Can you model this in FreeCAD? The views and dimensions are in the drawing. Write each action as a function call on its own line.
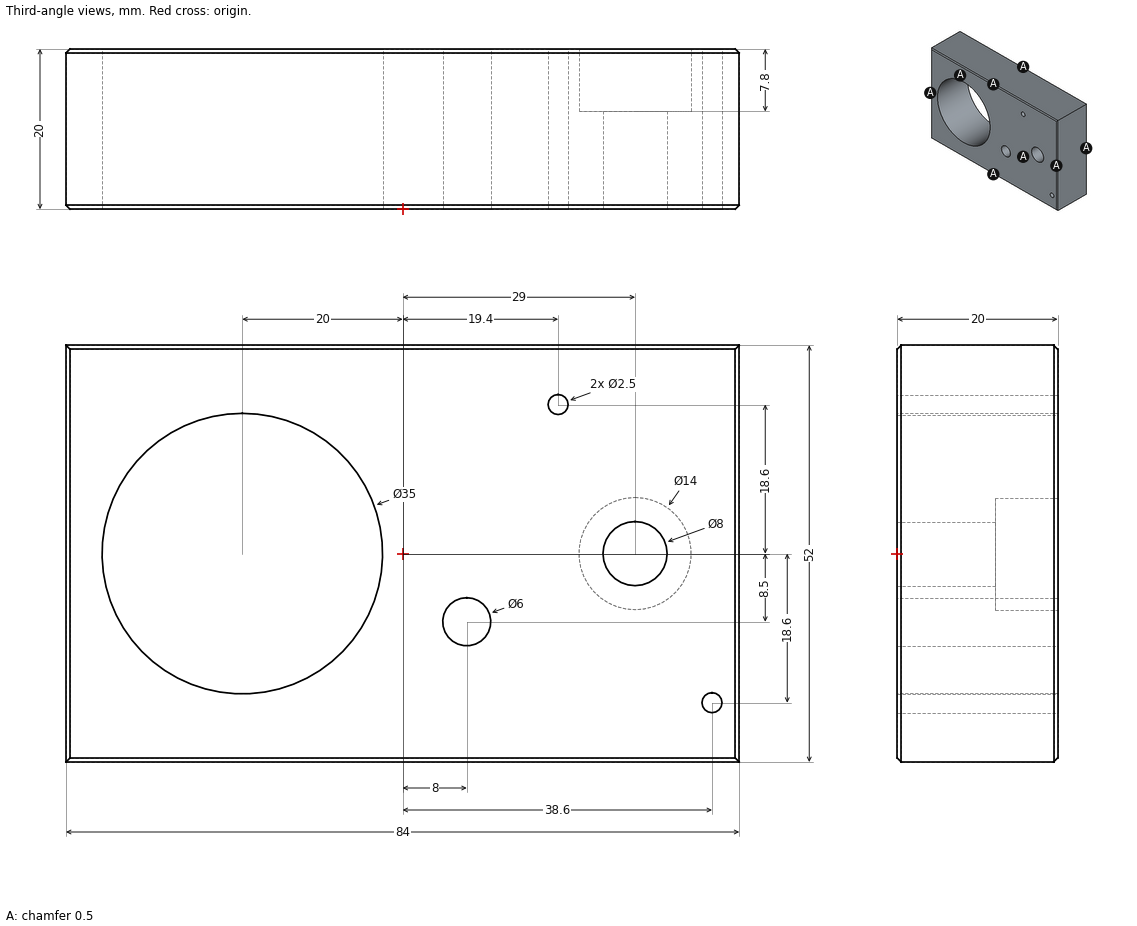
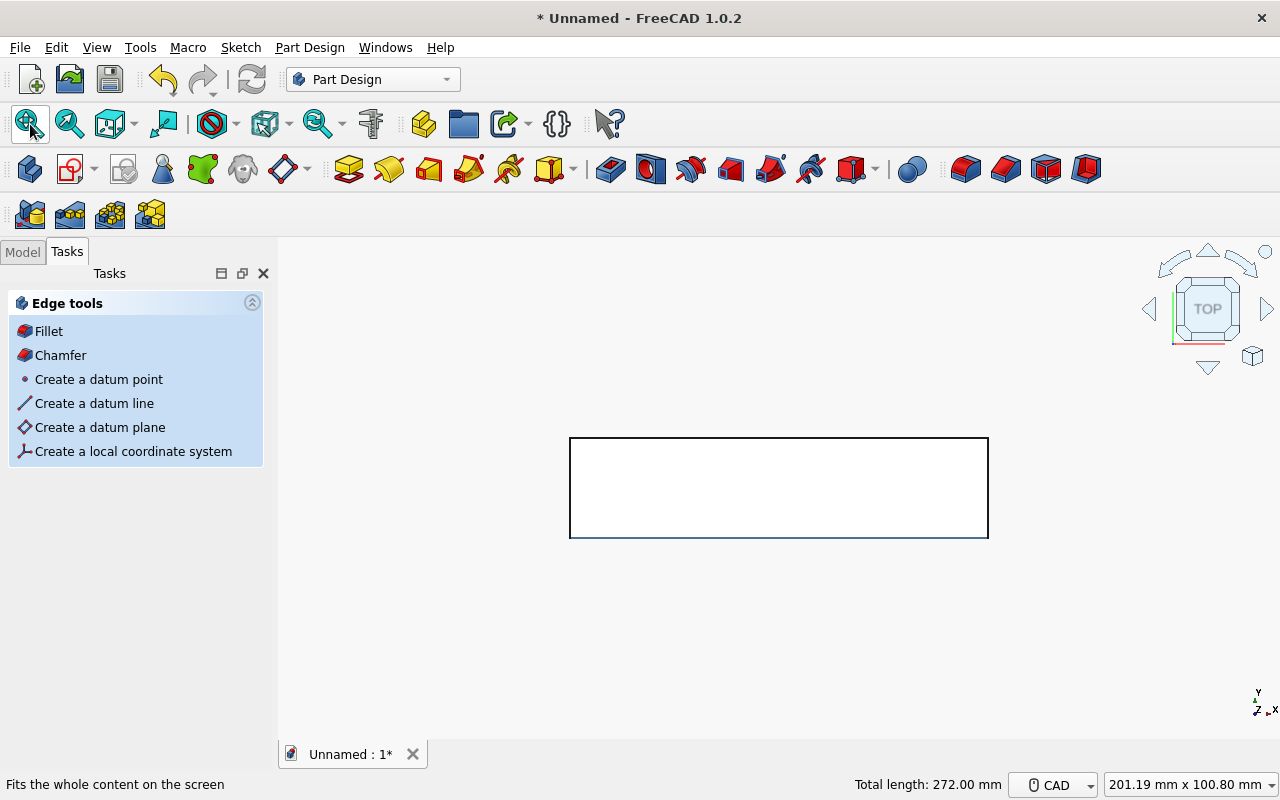
click(779, 437, ctrl)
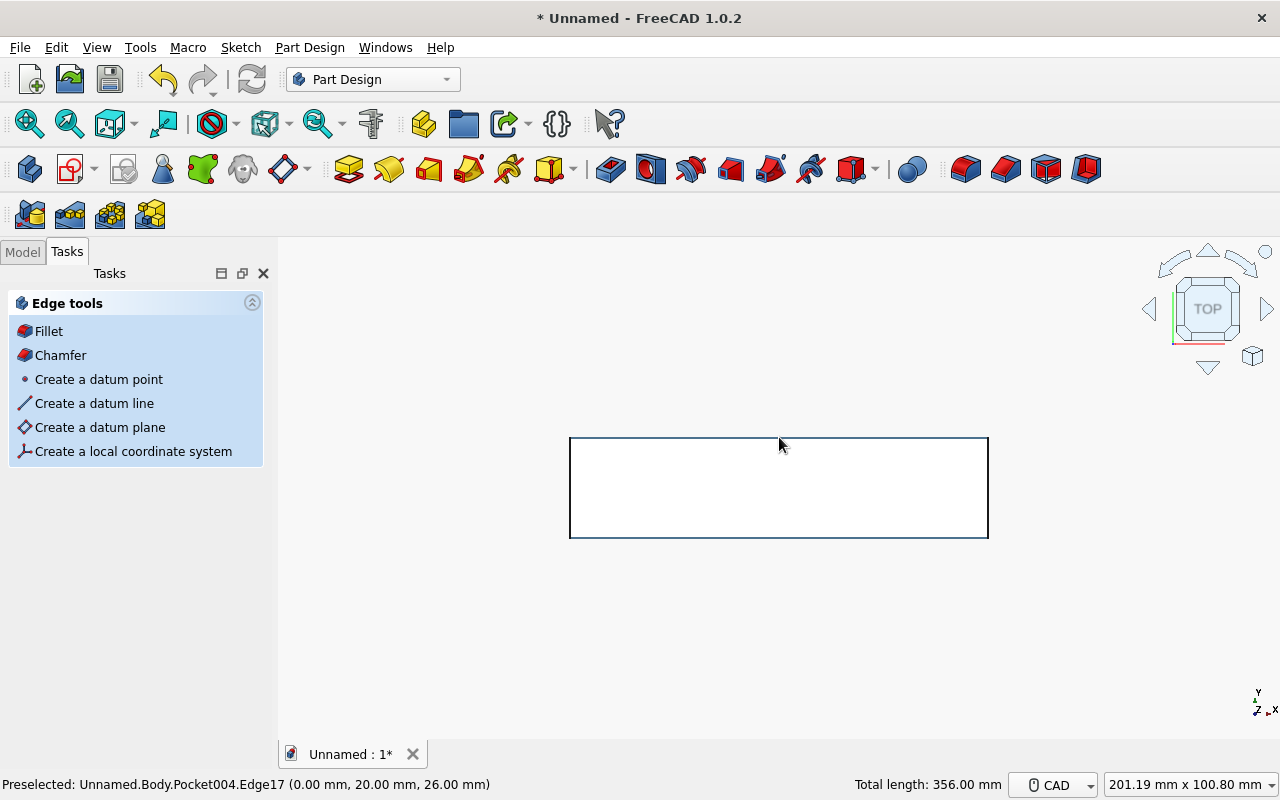
key(1)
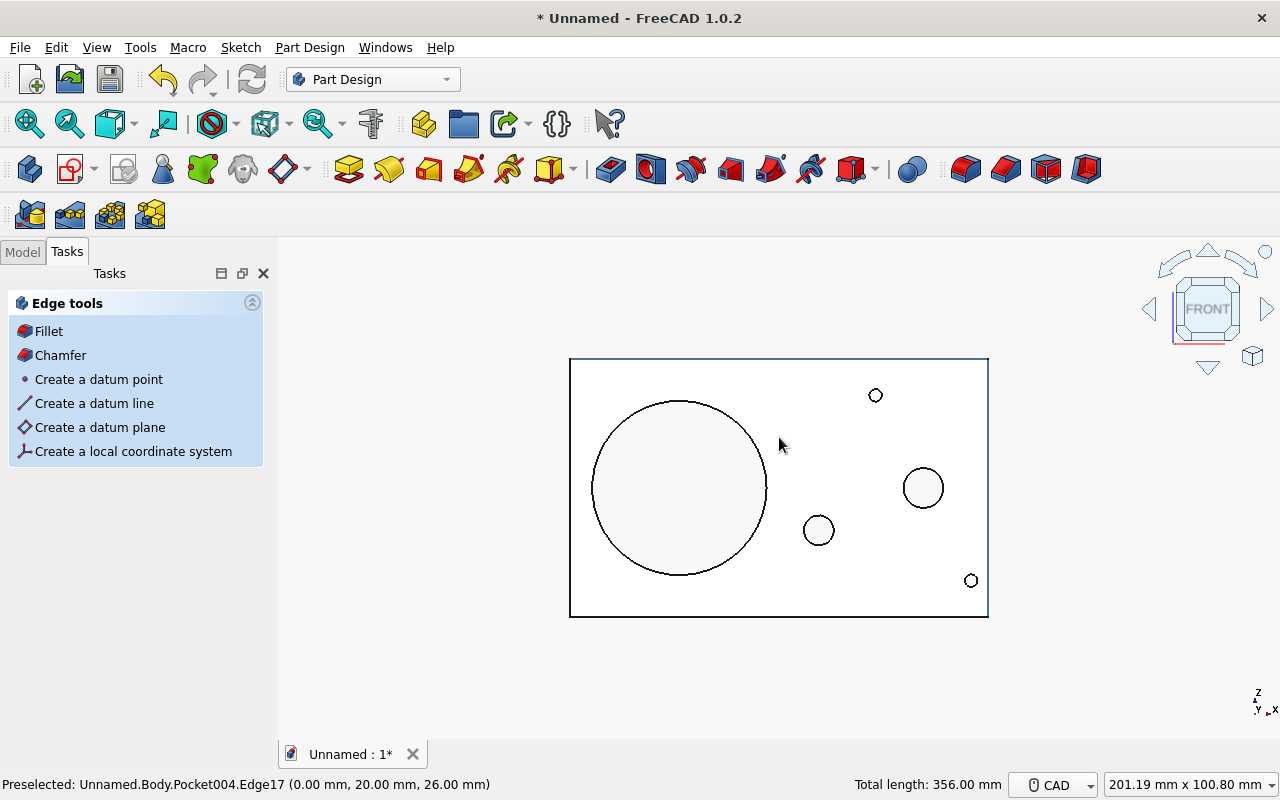
click(570, 487, ctrl)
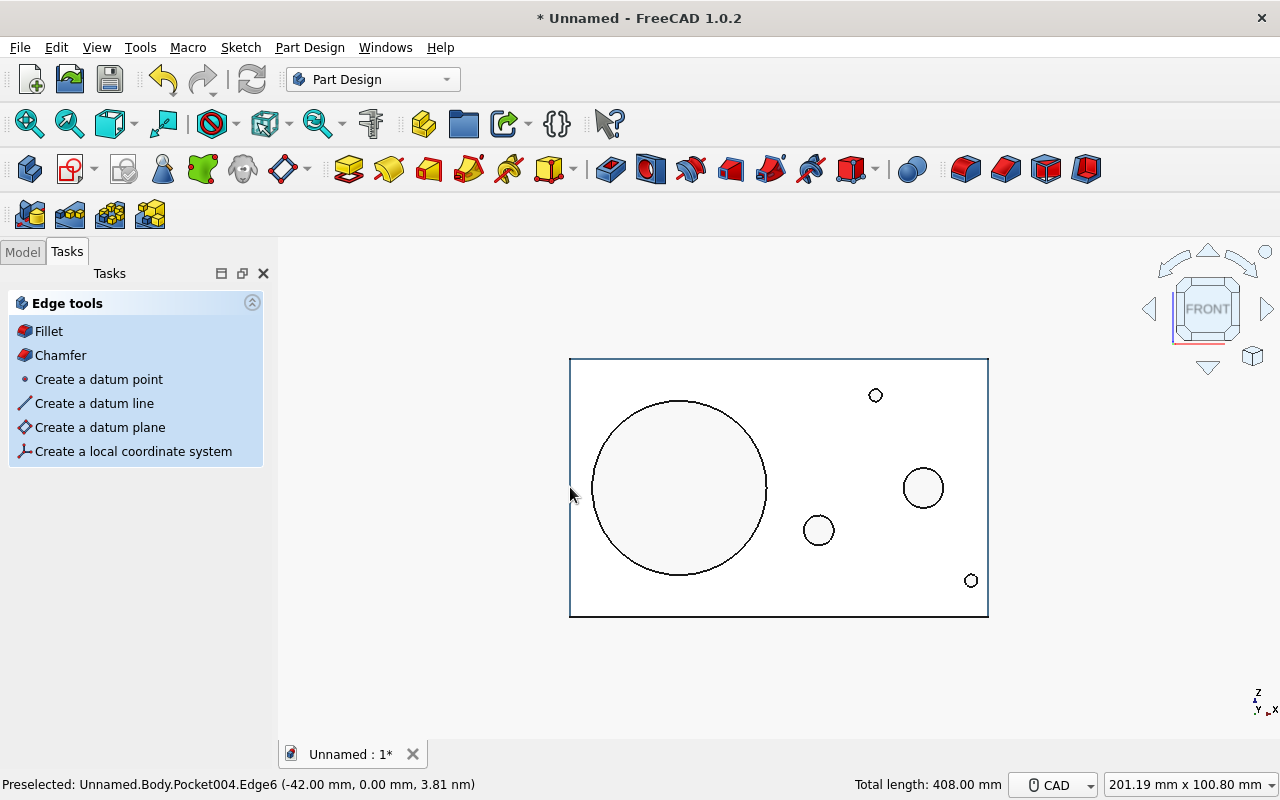
key(3)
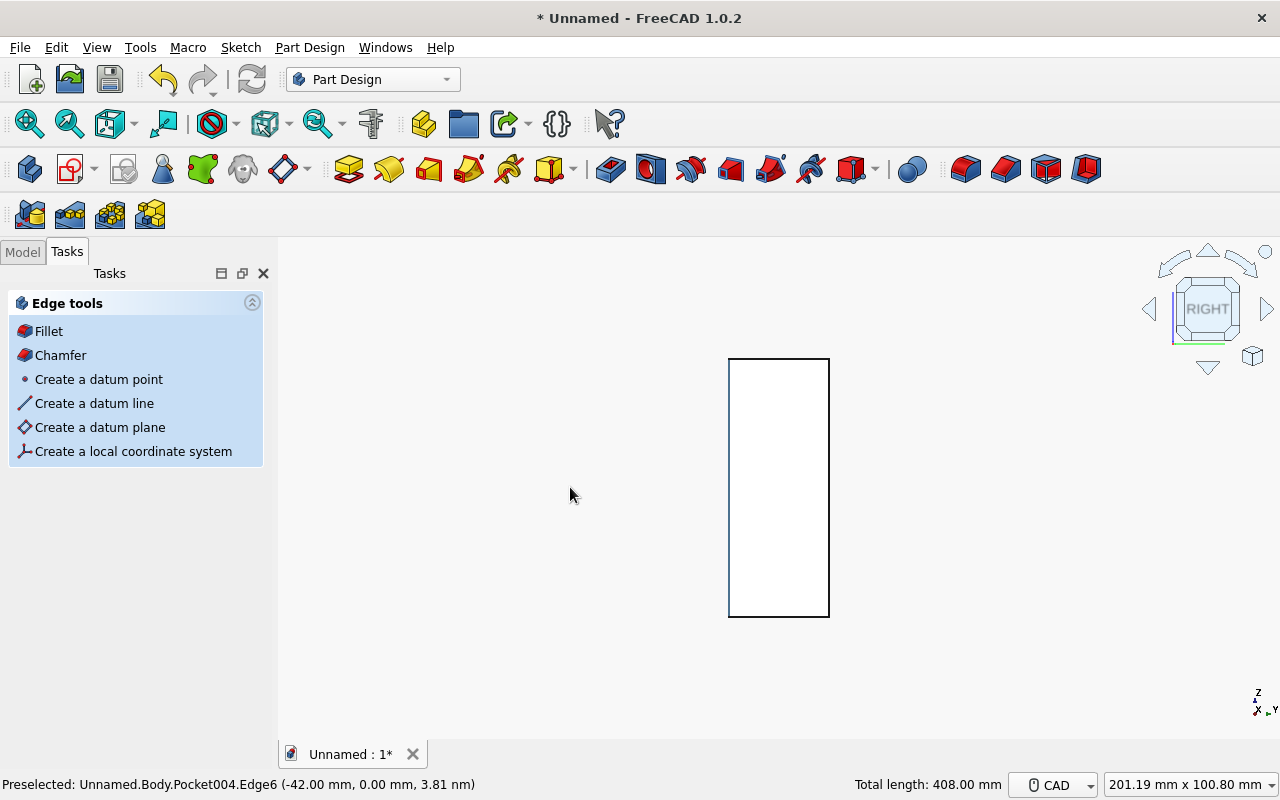
click(829, 487, ctrl)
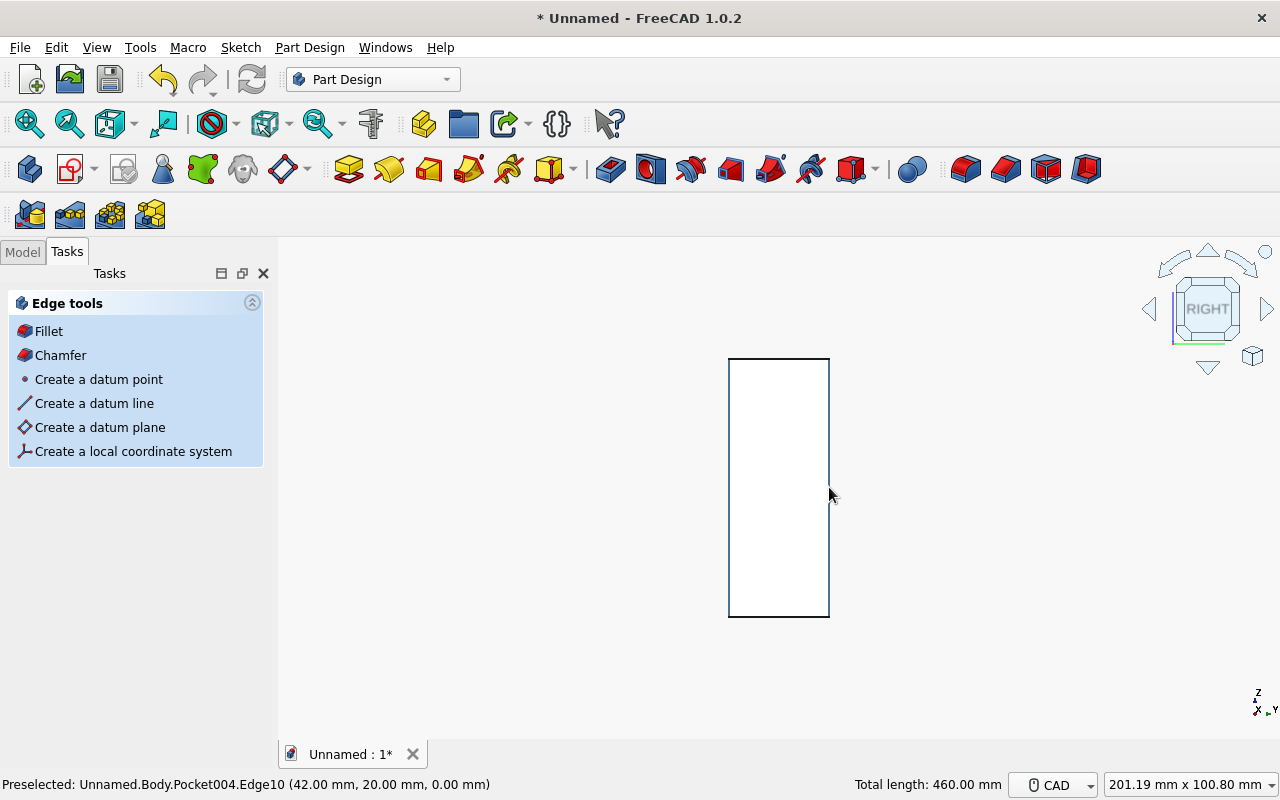
key(5)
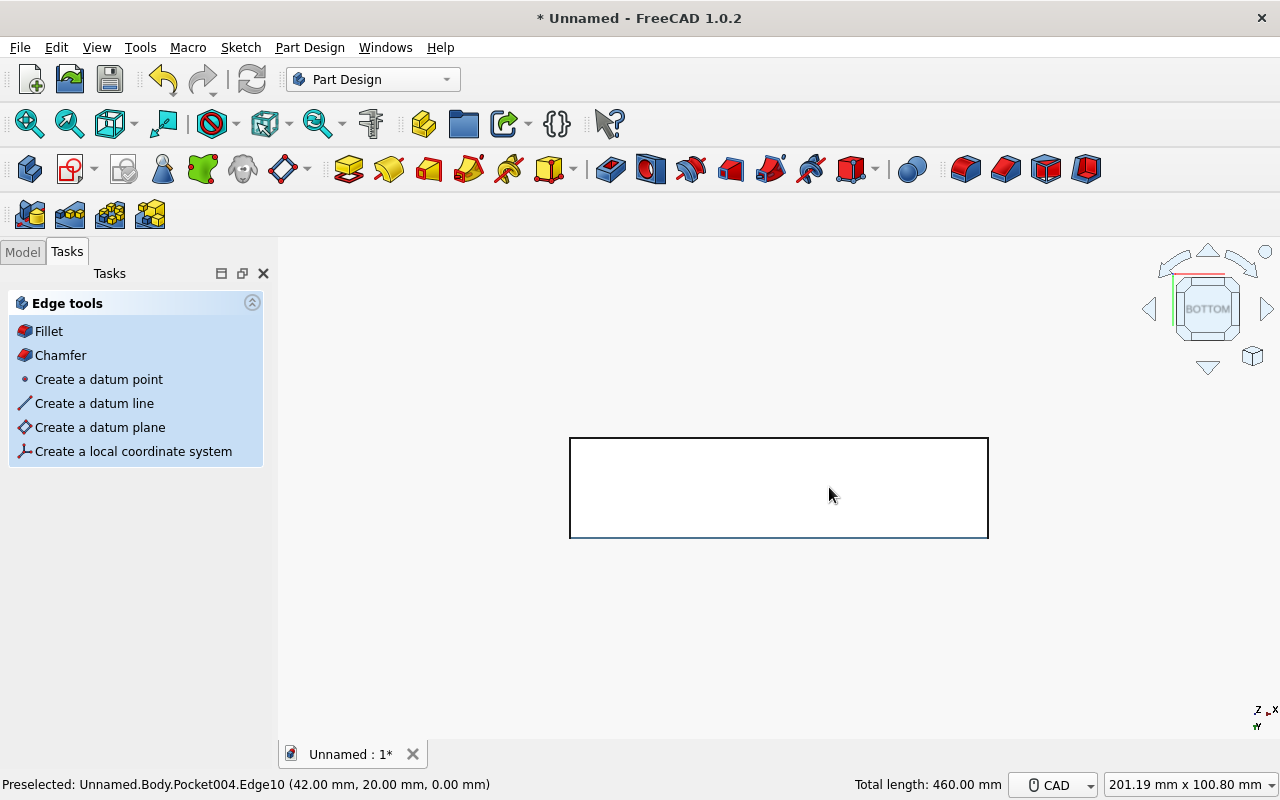
click(30, 124)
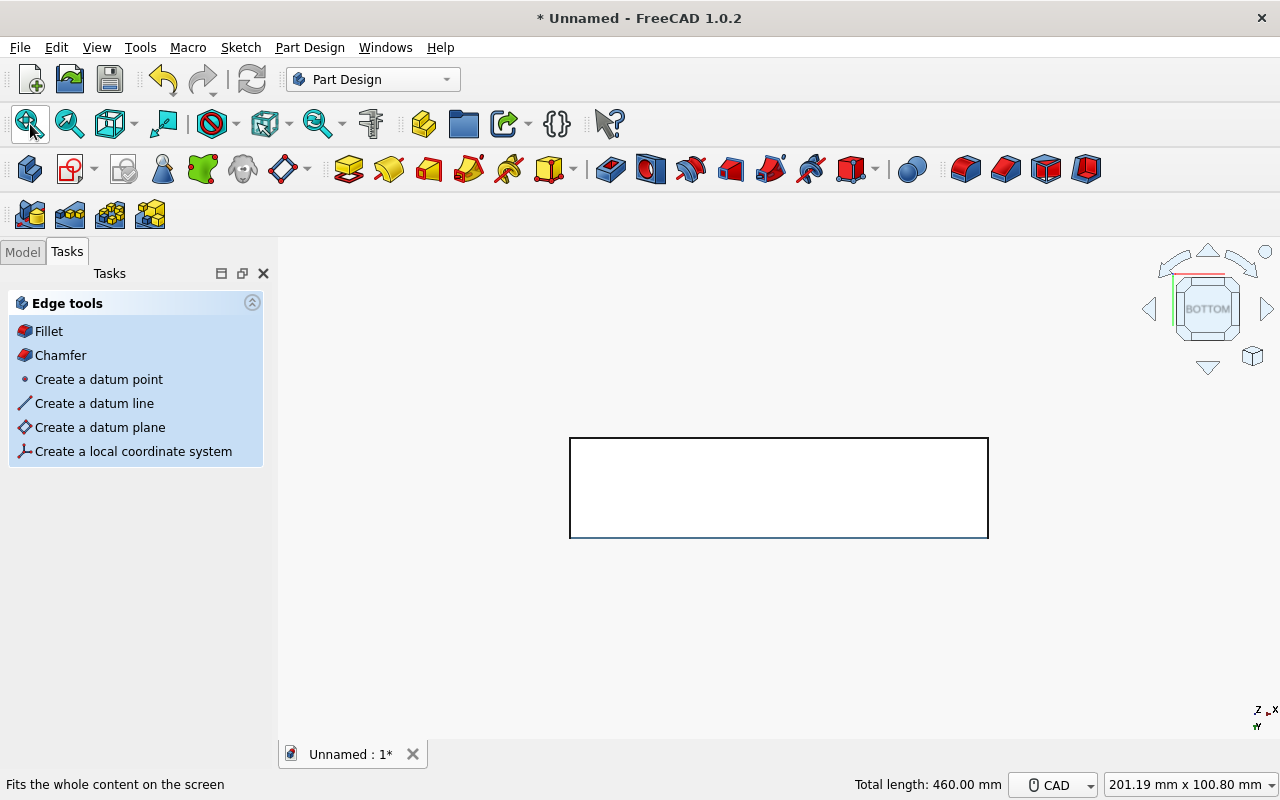
click(779, 437, ctrl)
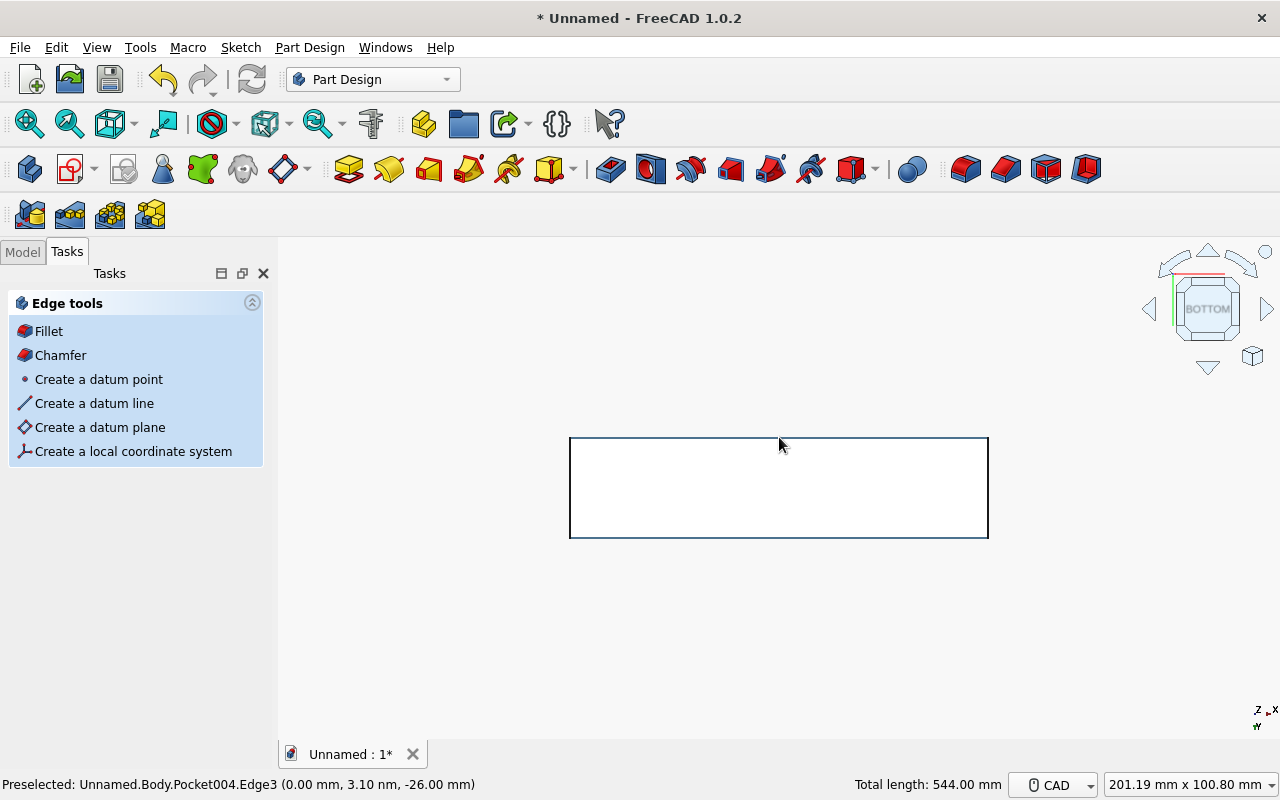
click(1006, 170)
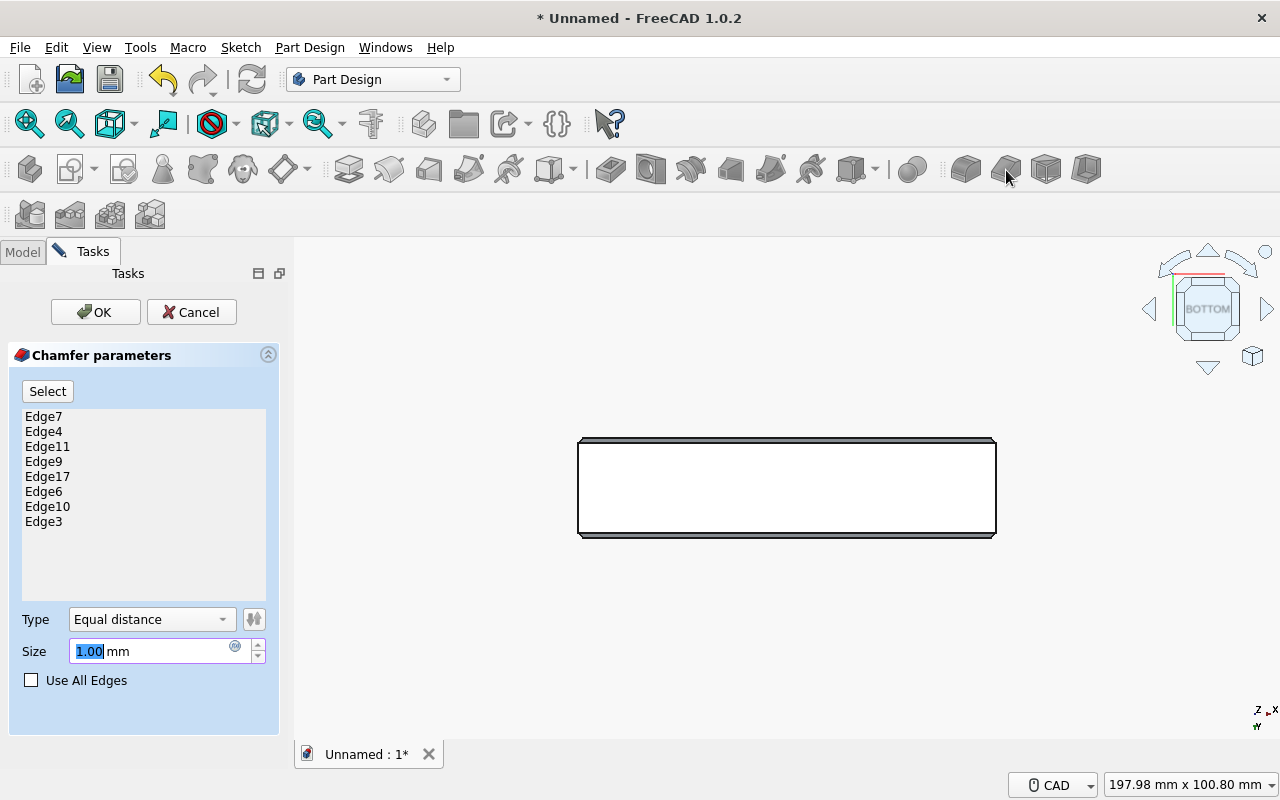
text(0.5)
key(Tab)